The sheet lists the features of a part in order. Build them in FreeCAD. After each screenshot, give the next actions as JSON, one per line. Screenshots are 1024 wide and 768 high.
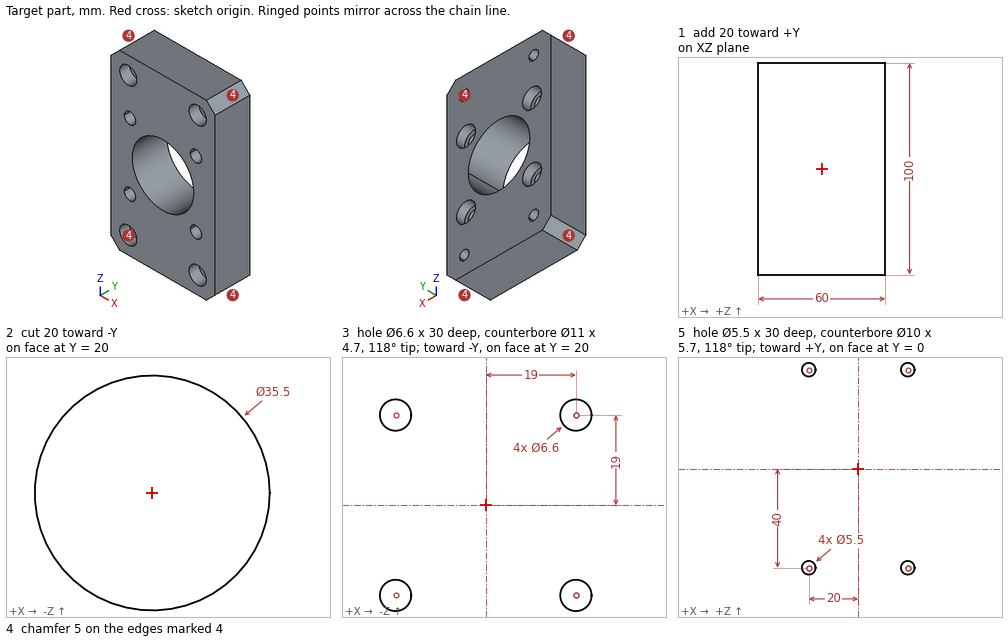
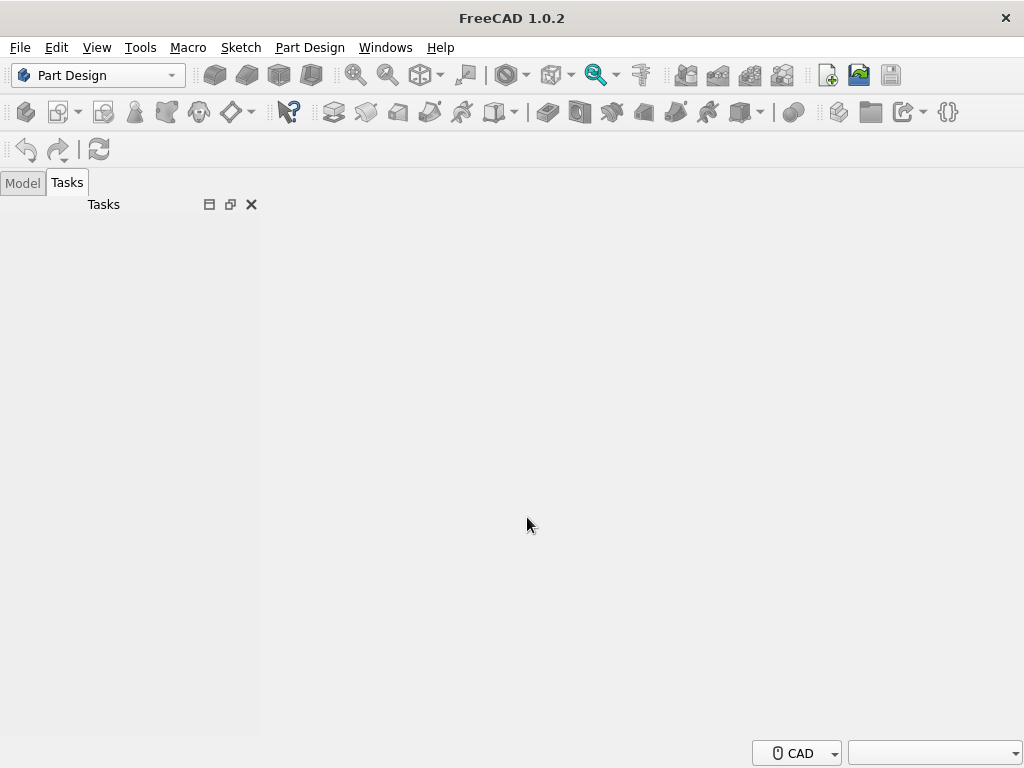
{"action": "left_click", "coordinate": [828, 76]}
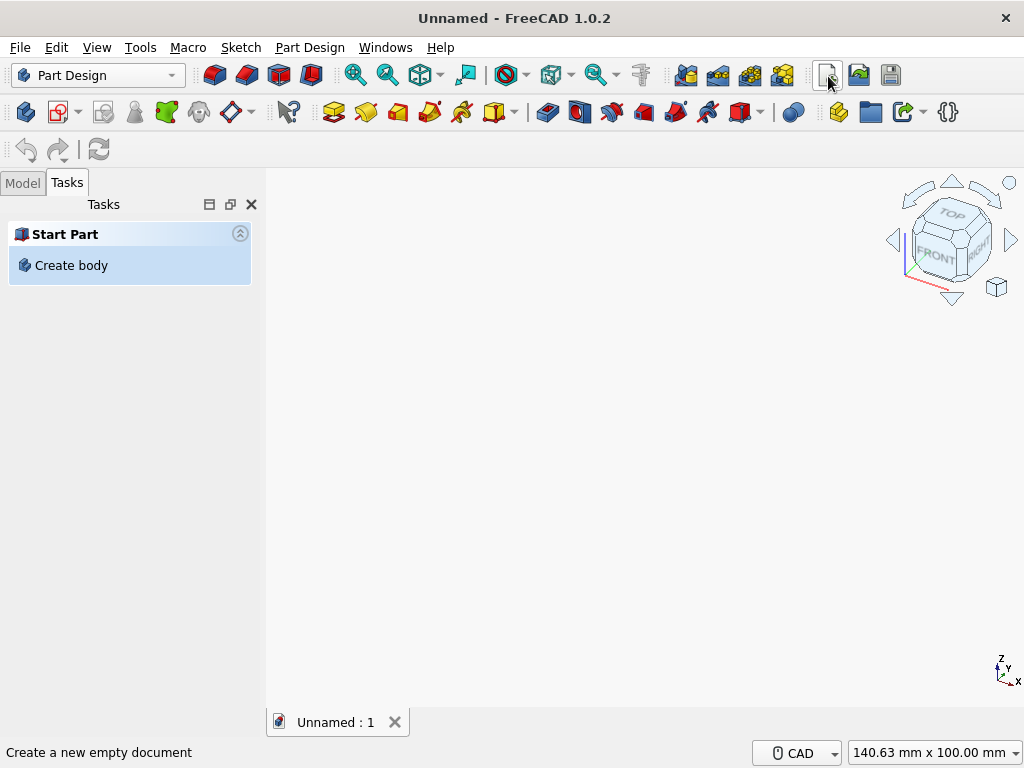
{"action": "left_click", "coordinate": [58, 112]}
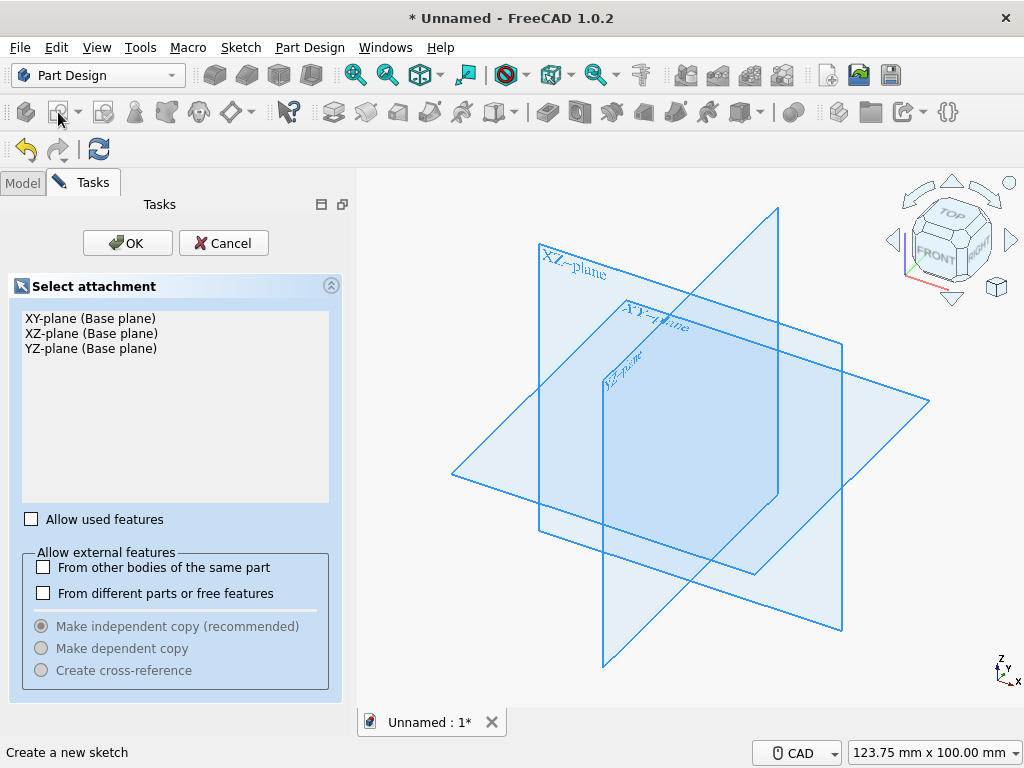
{"action": "left_click", "coordinate": [82, 334]}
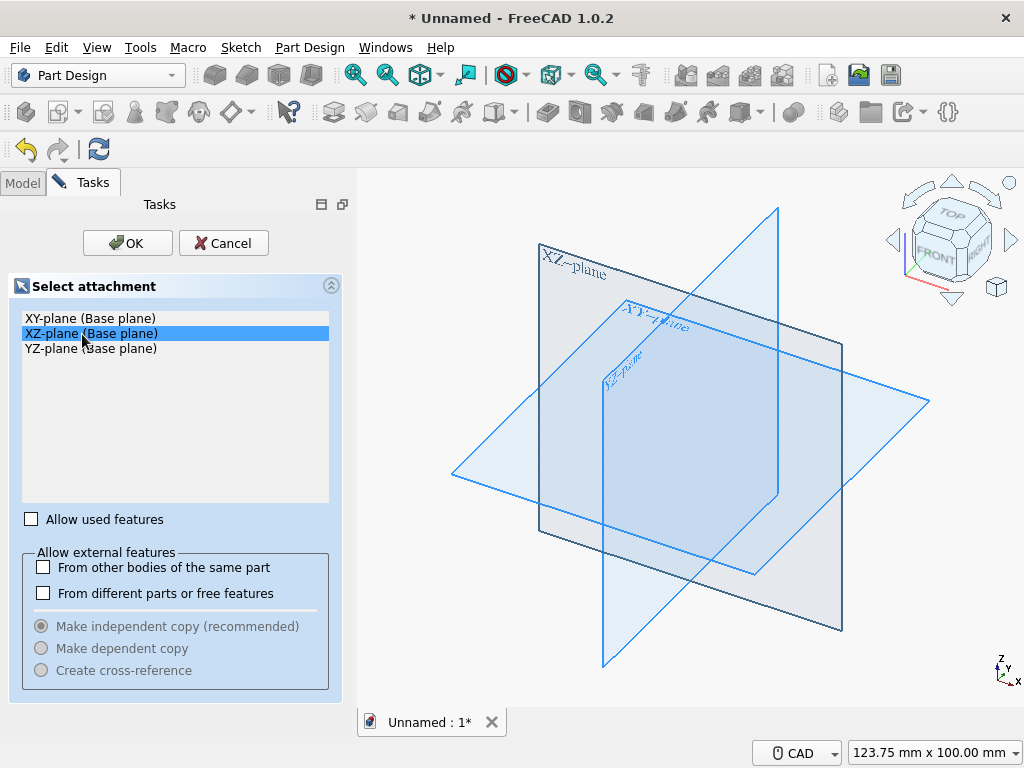
{"action": "left_click", "coordinate": [128, 243]}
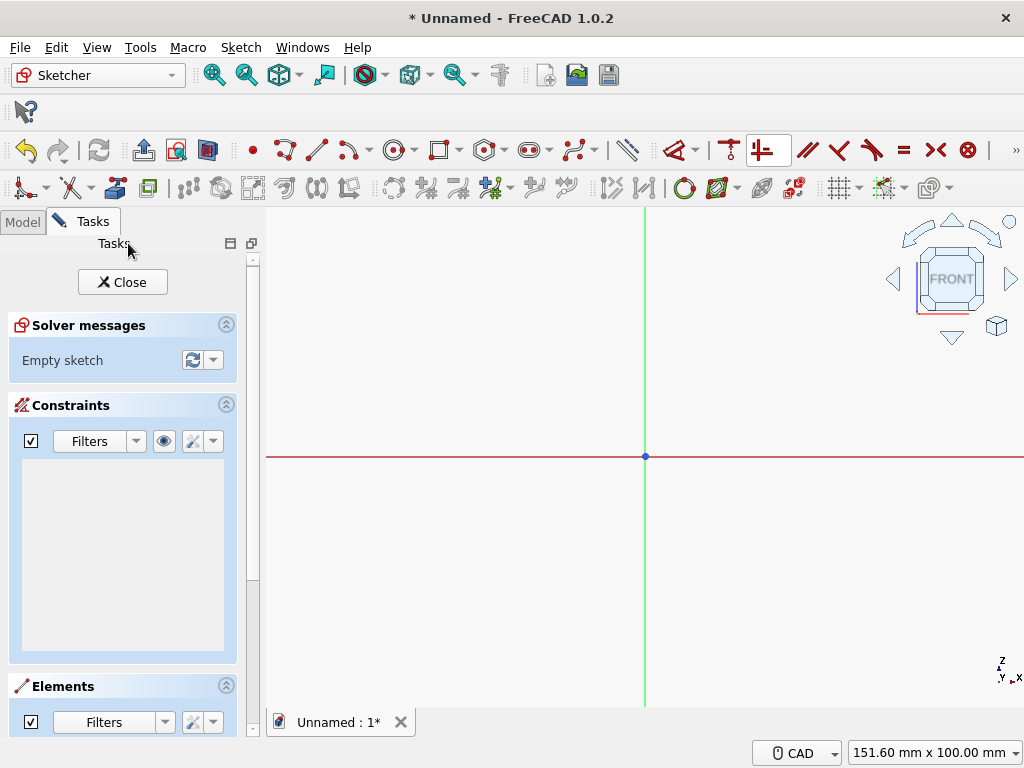
{"action": "scroll", "coordinate": [437, 457], "scroll_direction": "down", "scroll_amount": 2}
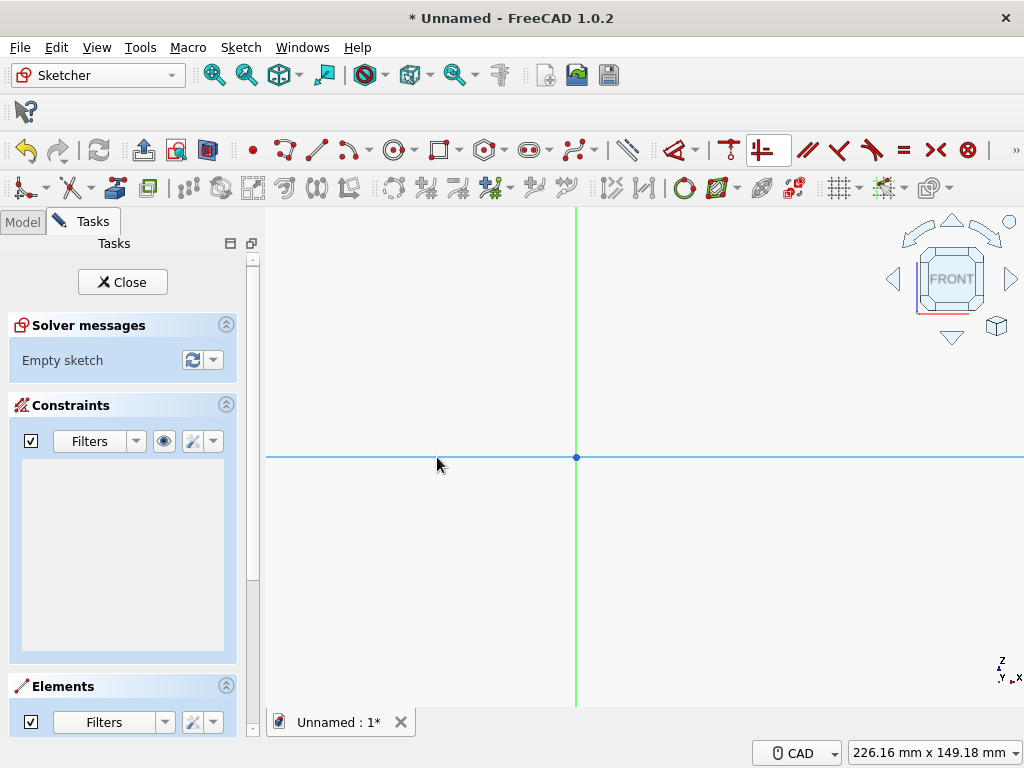
{"action": "left_click", "coordinate": [462, 150]}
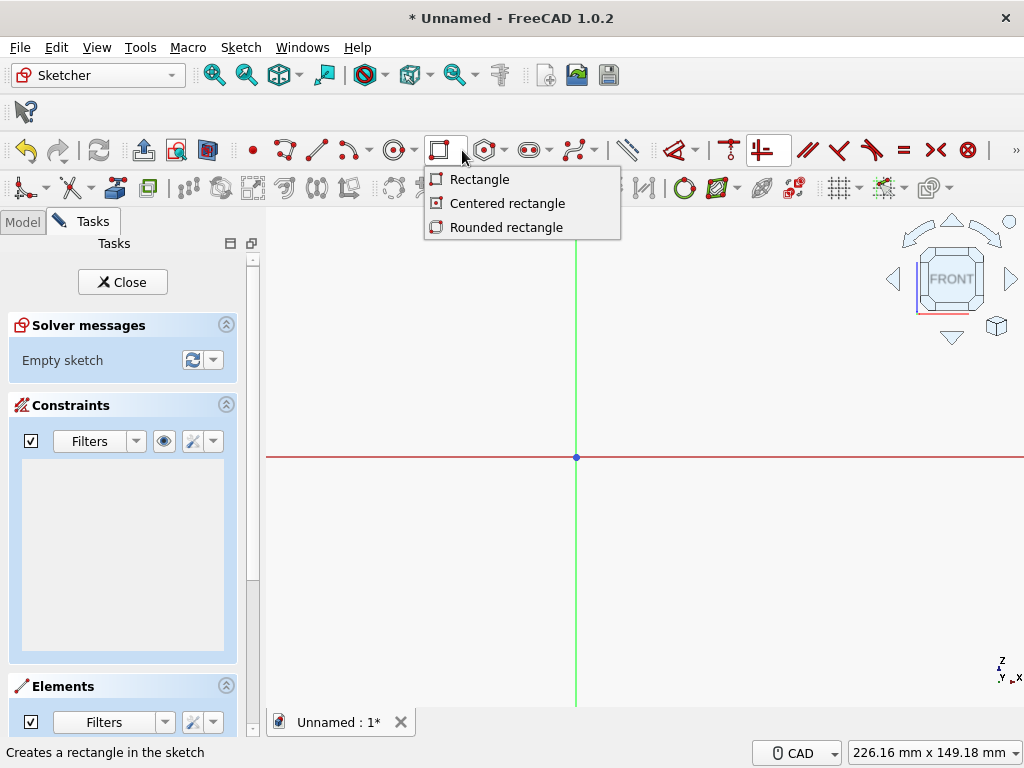
{"action": "left_click", "coordinate": [522, 203]}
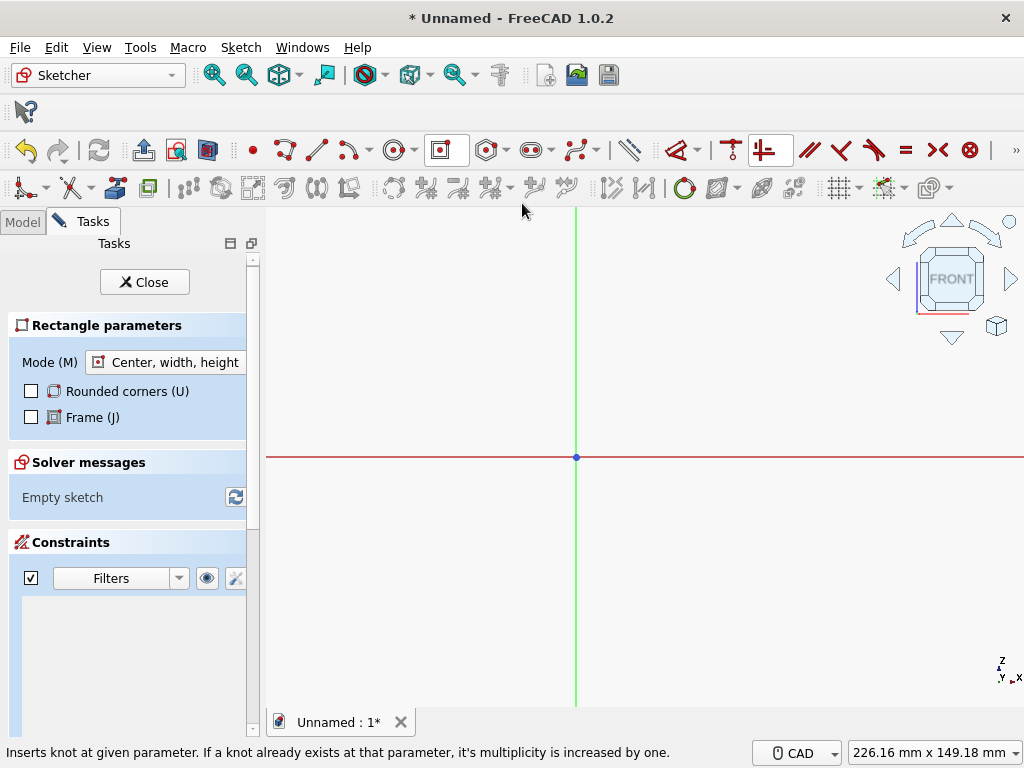
{"action": "left_click", "coordinate": [577, 457]}
{"action": "left_click", "coordinate": [677, 290]}
{"action": "key", "text": "Escape"}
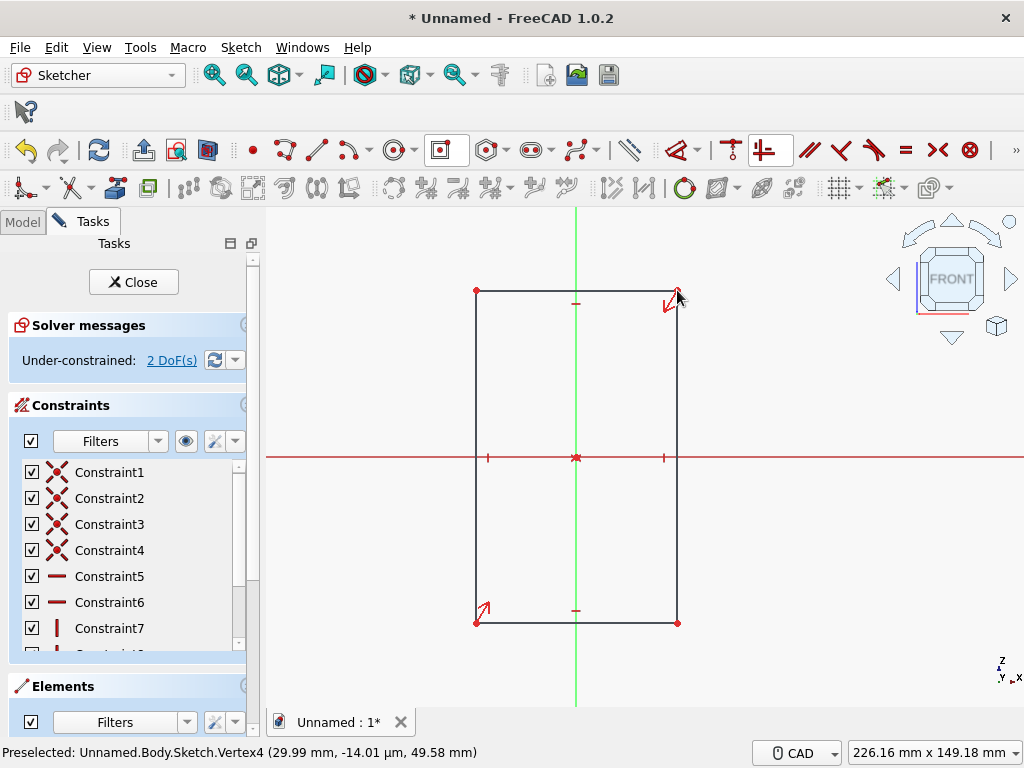
{"action": "left_click", "coordinate": [676, 150]}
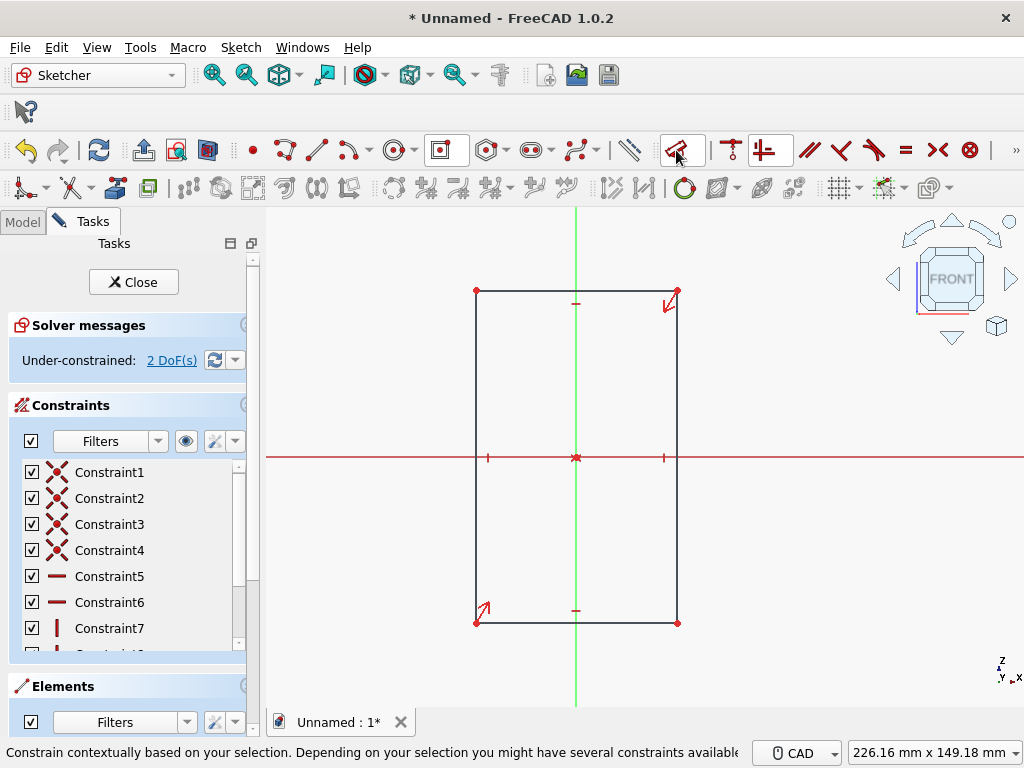
{"action": "left_click", "coordinate": [536, 623]}
{"action": "left_click", "coordinate": [530, 657]}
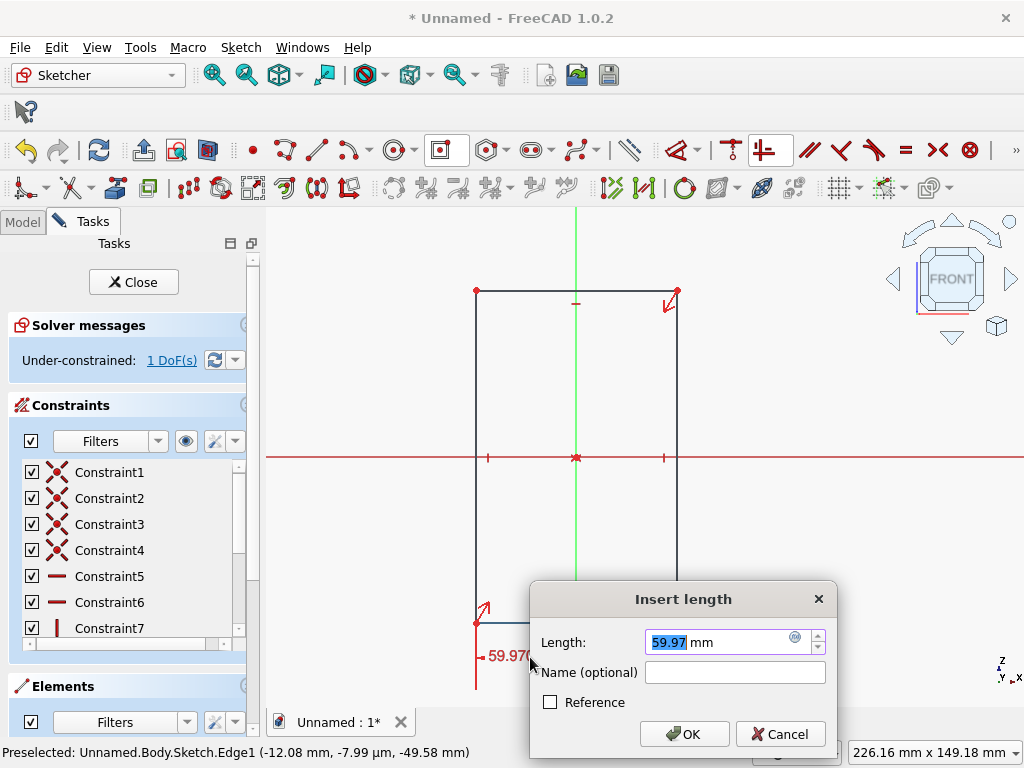
{"action": "type", "text": "60"}
{"action": "key", "text": "Return"}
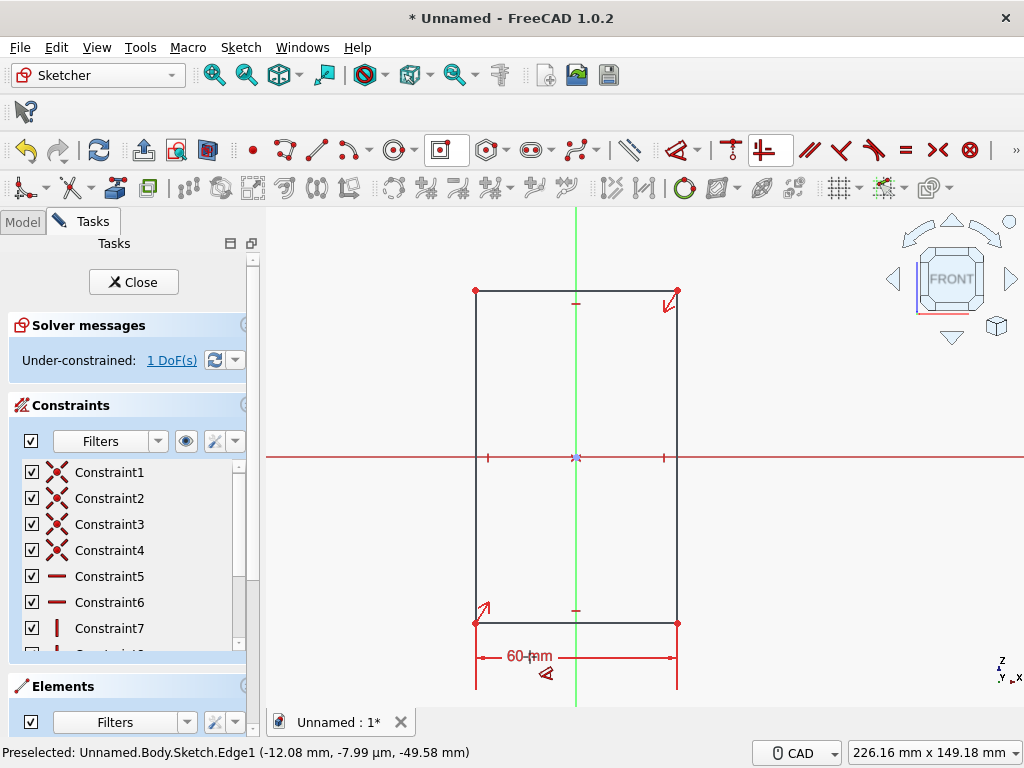
{"action": "left_click", "coordinate": [677, 524]}
{"action": "left_click", "coordinate": [711, 381]}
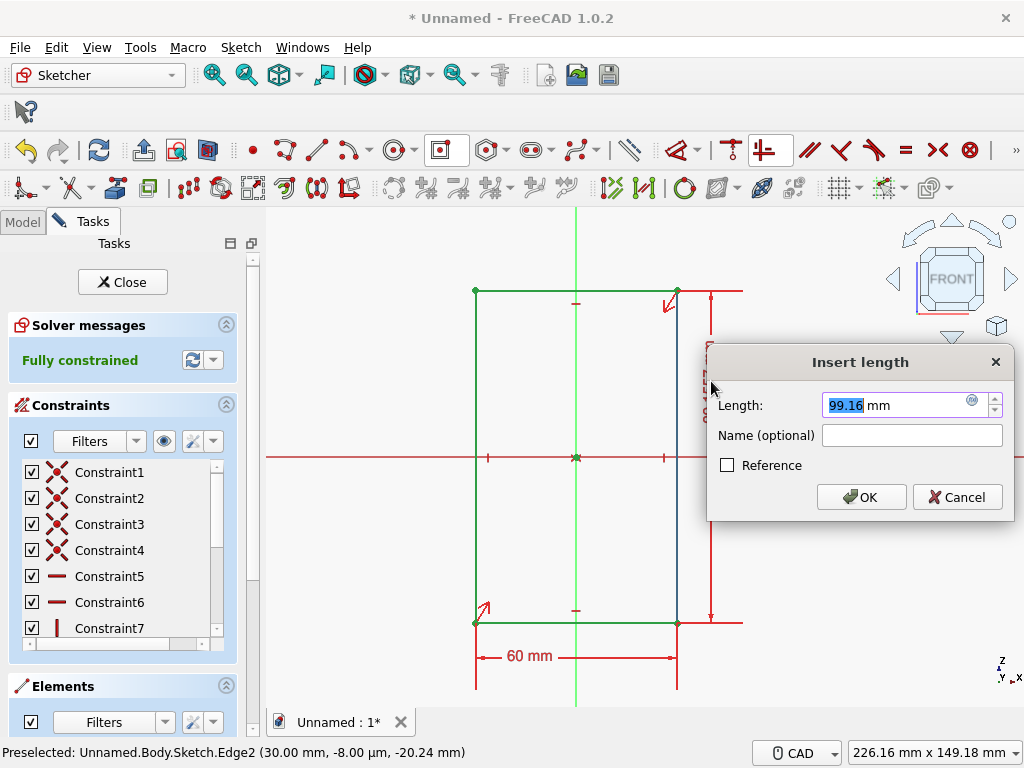
{"action": "type", "text": "100"}
{"action": "key", "text": "Return"}
{"action": "key", "text": "Escape"}